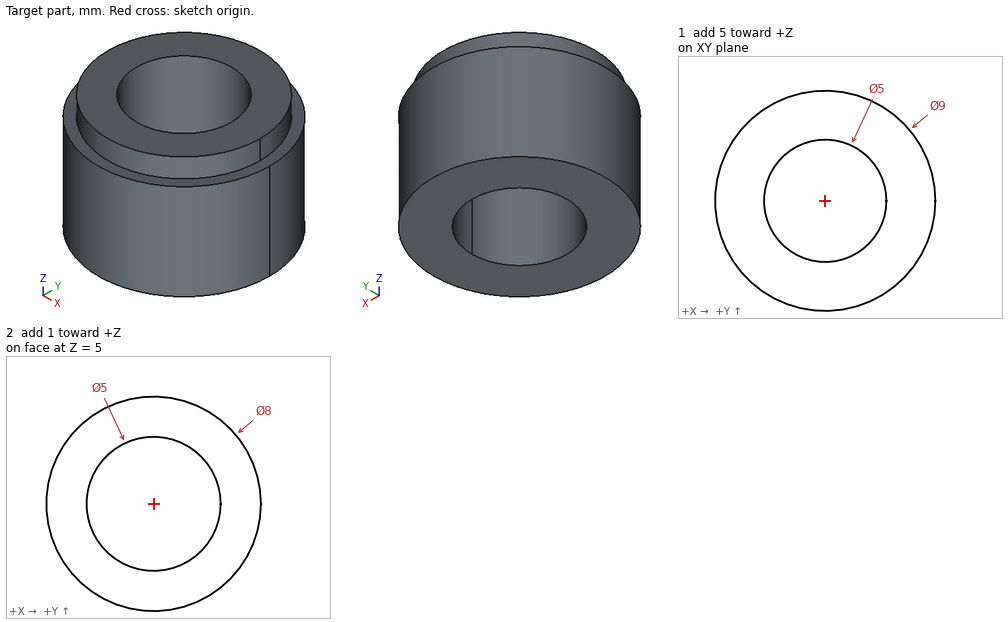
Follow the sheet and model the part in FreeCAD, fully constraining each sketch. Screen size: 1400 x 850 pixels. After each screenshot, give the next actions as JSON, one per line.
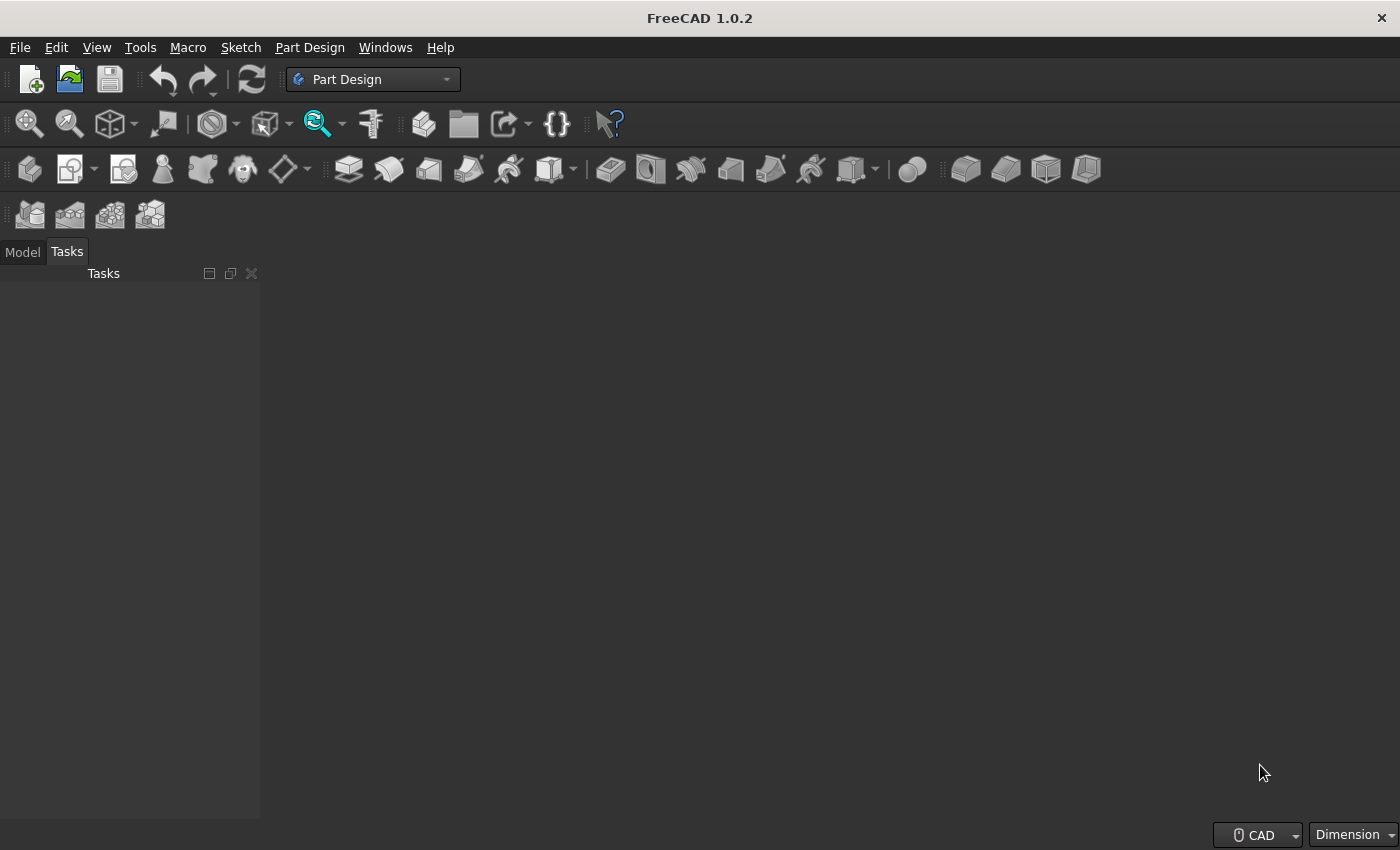
{"action": "left_click", "coordinate": [30, 80]}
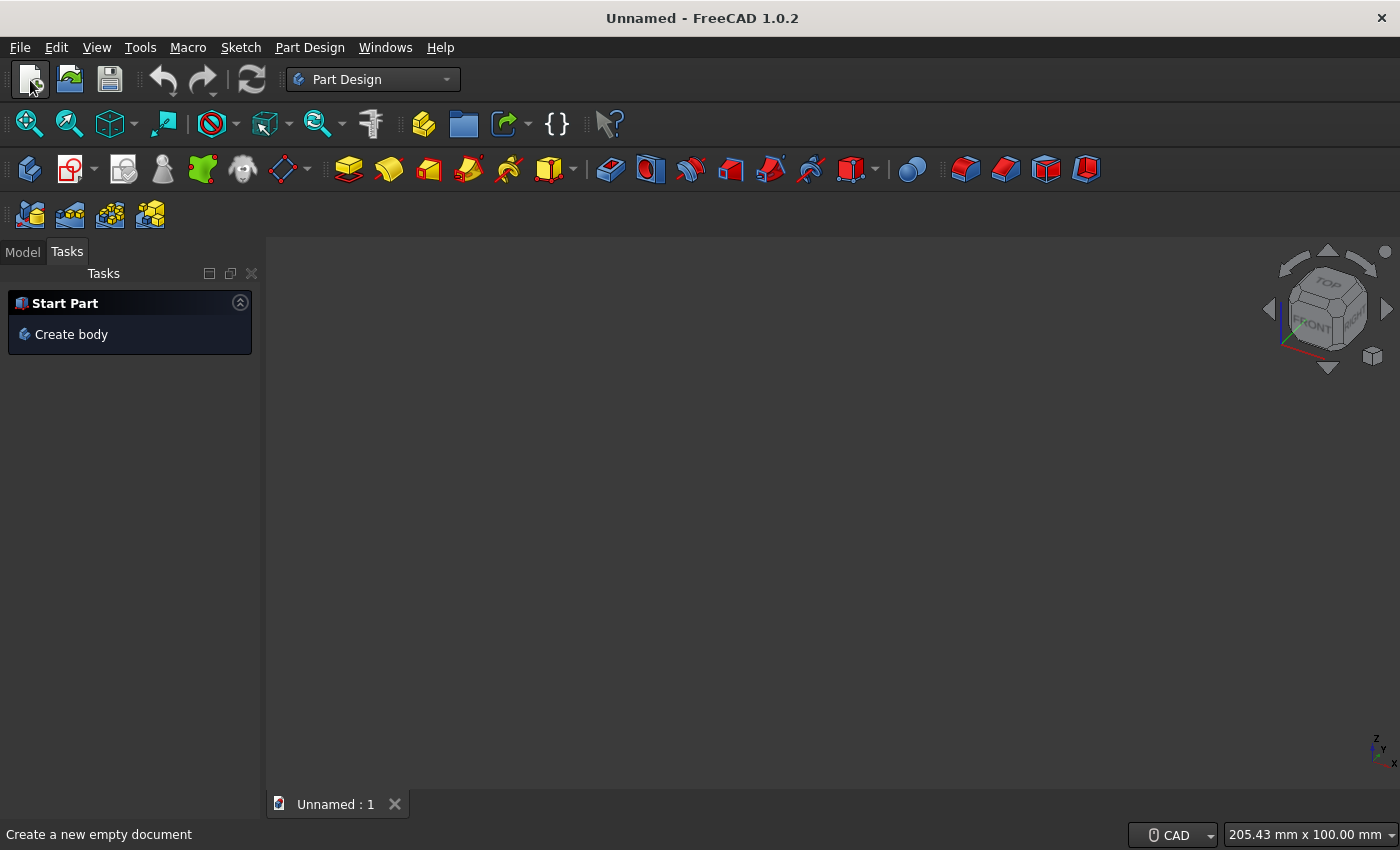
{"action": "left_click", "coordinate": [70, 170]}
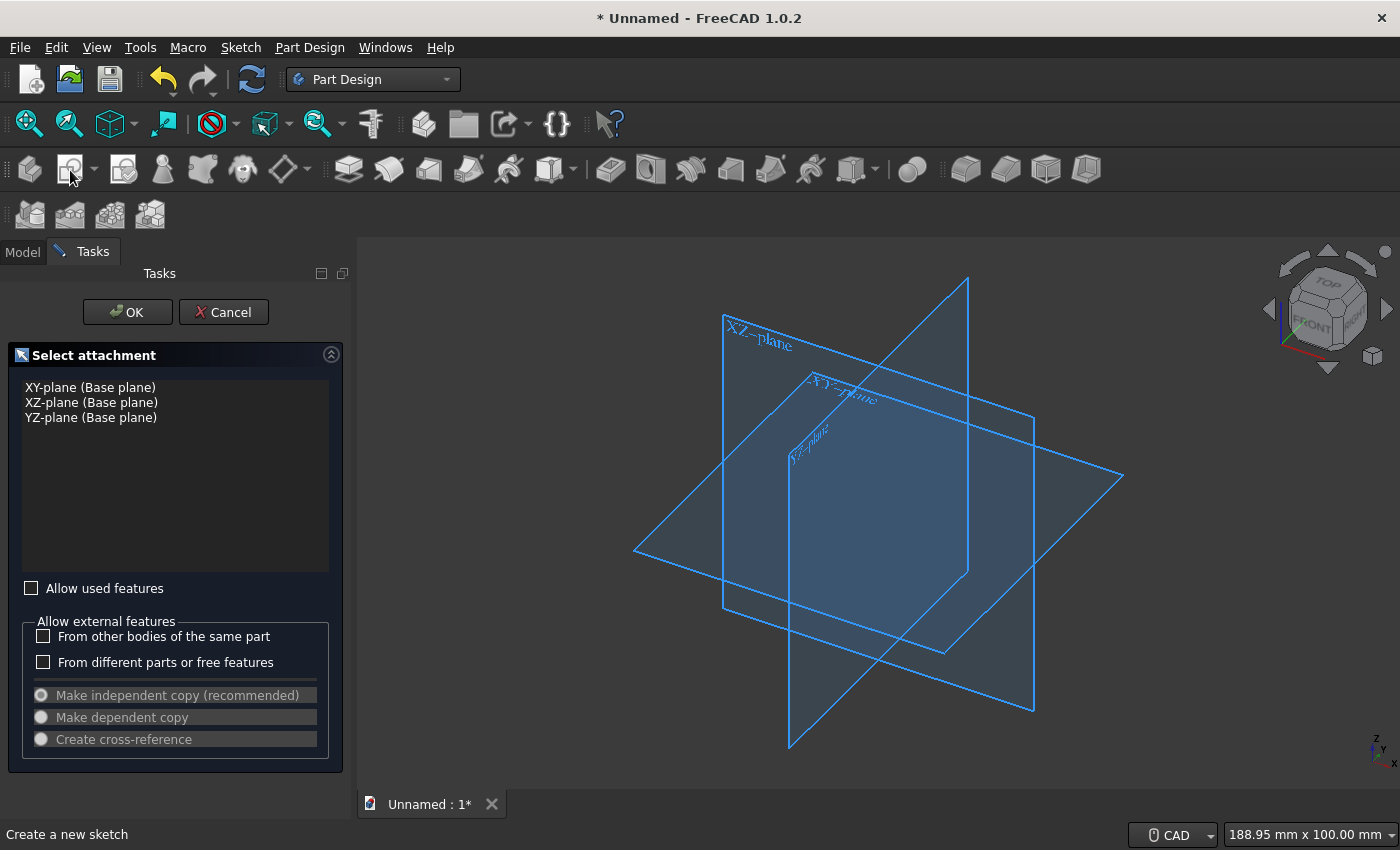
{"action": "left_click", "coordinate": [82, 388]}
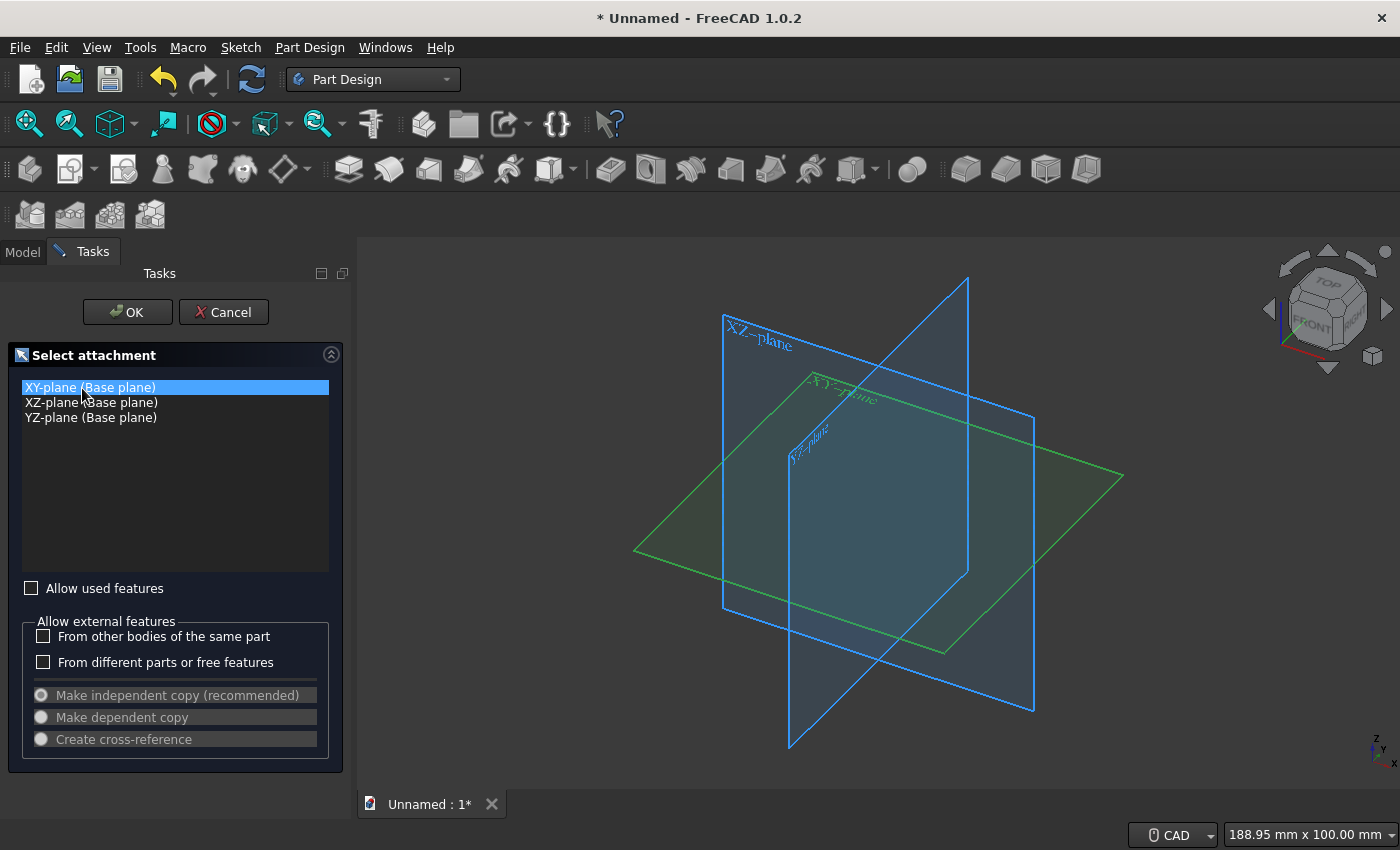
{"action": "left_click", "coordinate": [128, 312]}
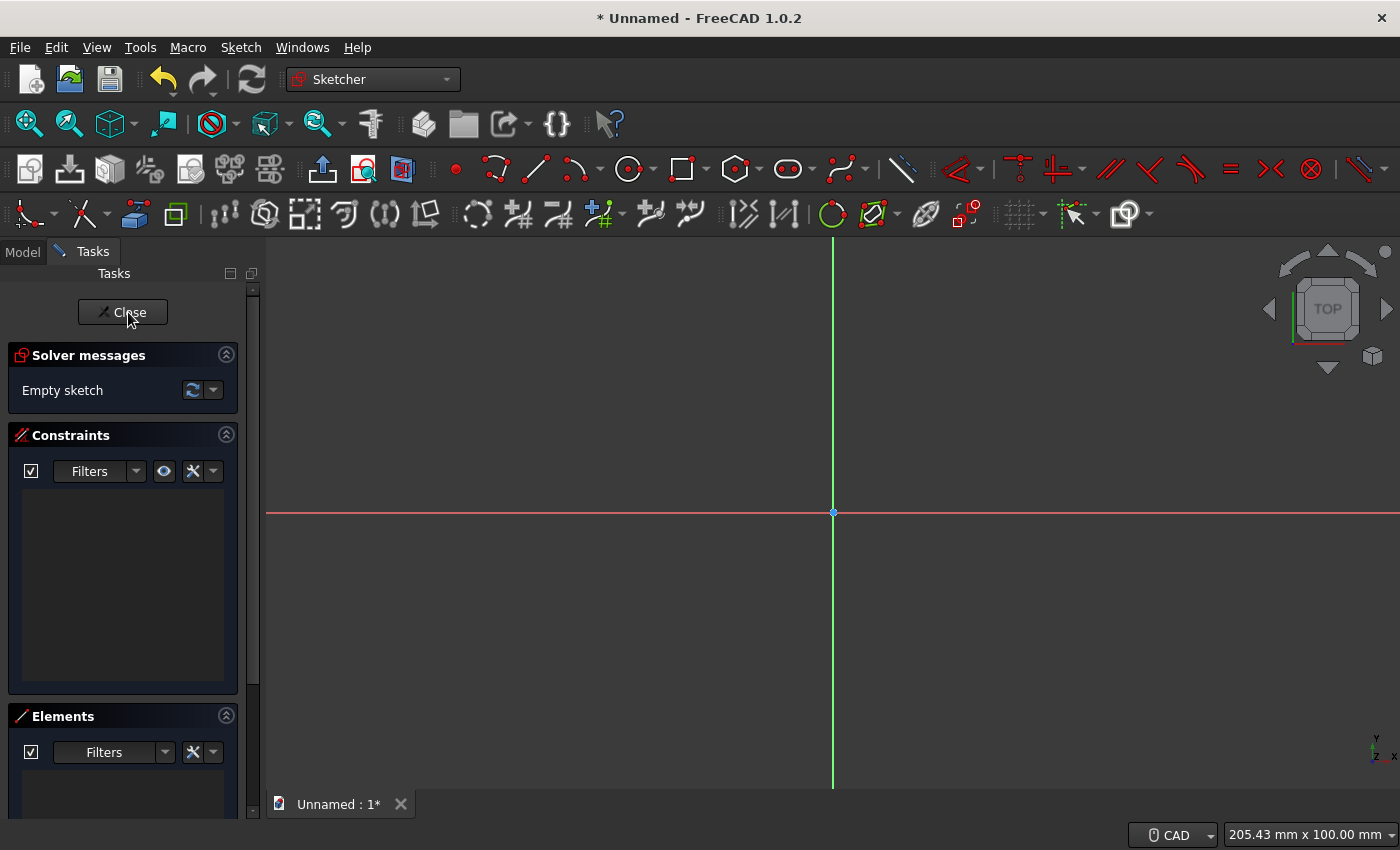
{"action": "scroll", "coordinate": [844, 513], "scroll_direction": "up", "scroll_amount": 10}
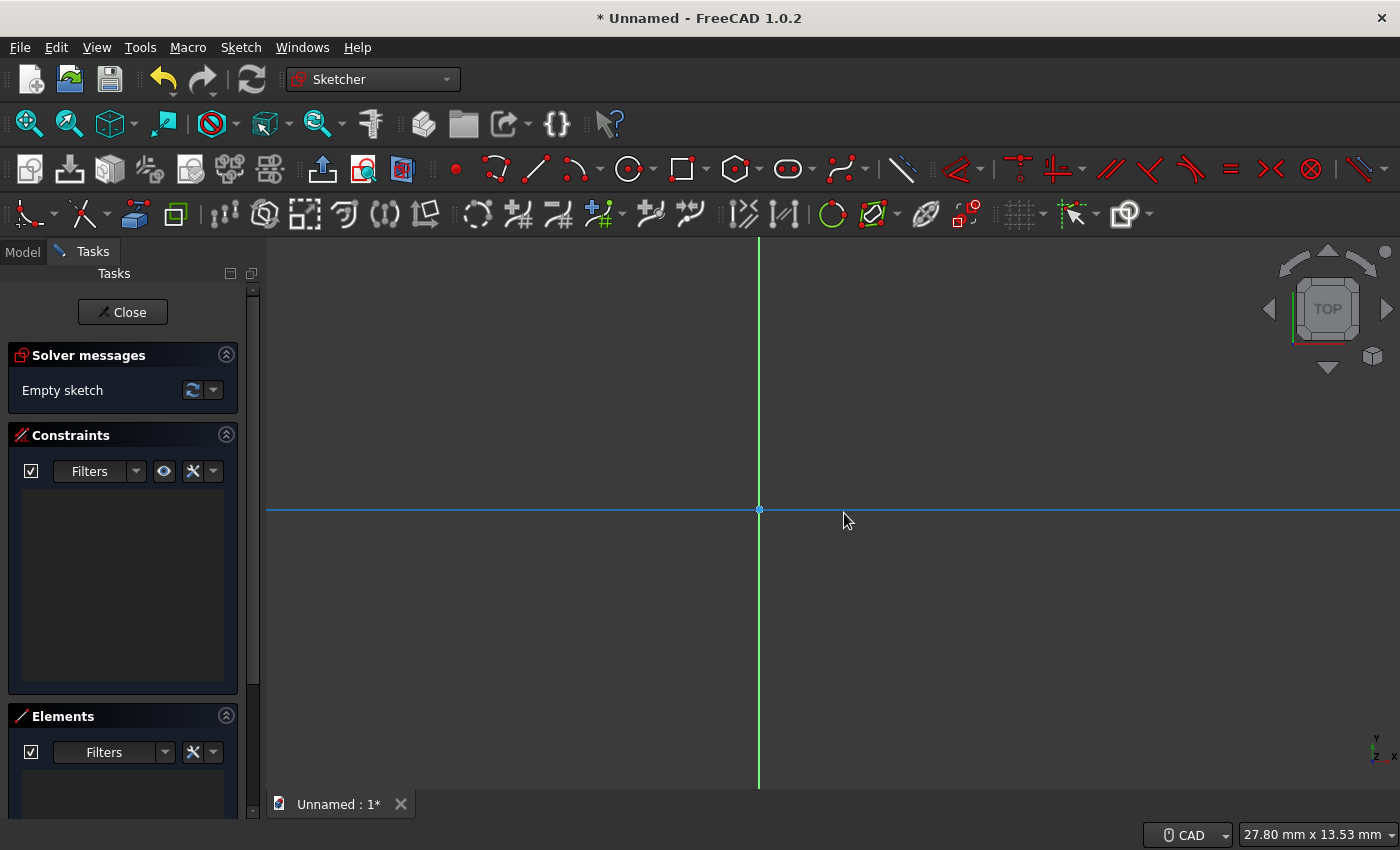
{"action": "left_click", "coordinate": [630, 170]}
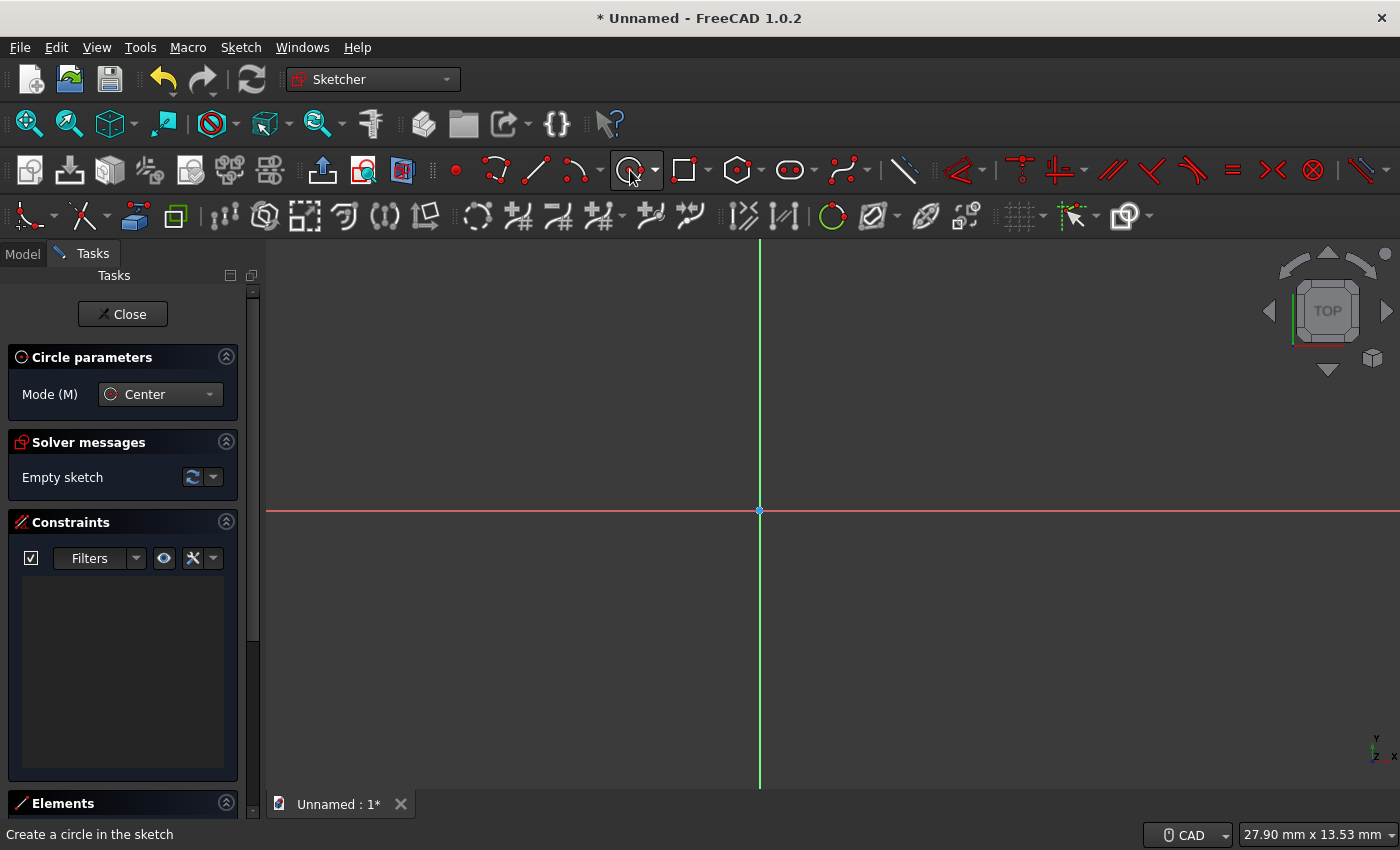
{"action": "left_click", "coordinate": [760, 511]}
{"action": "left_click", "coordinate": [889, 381]}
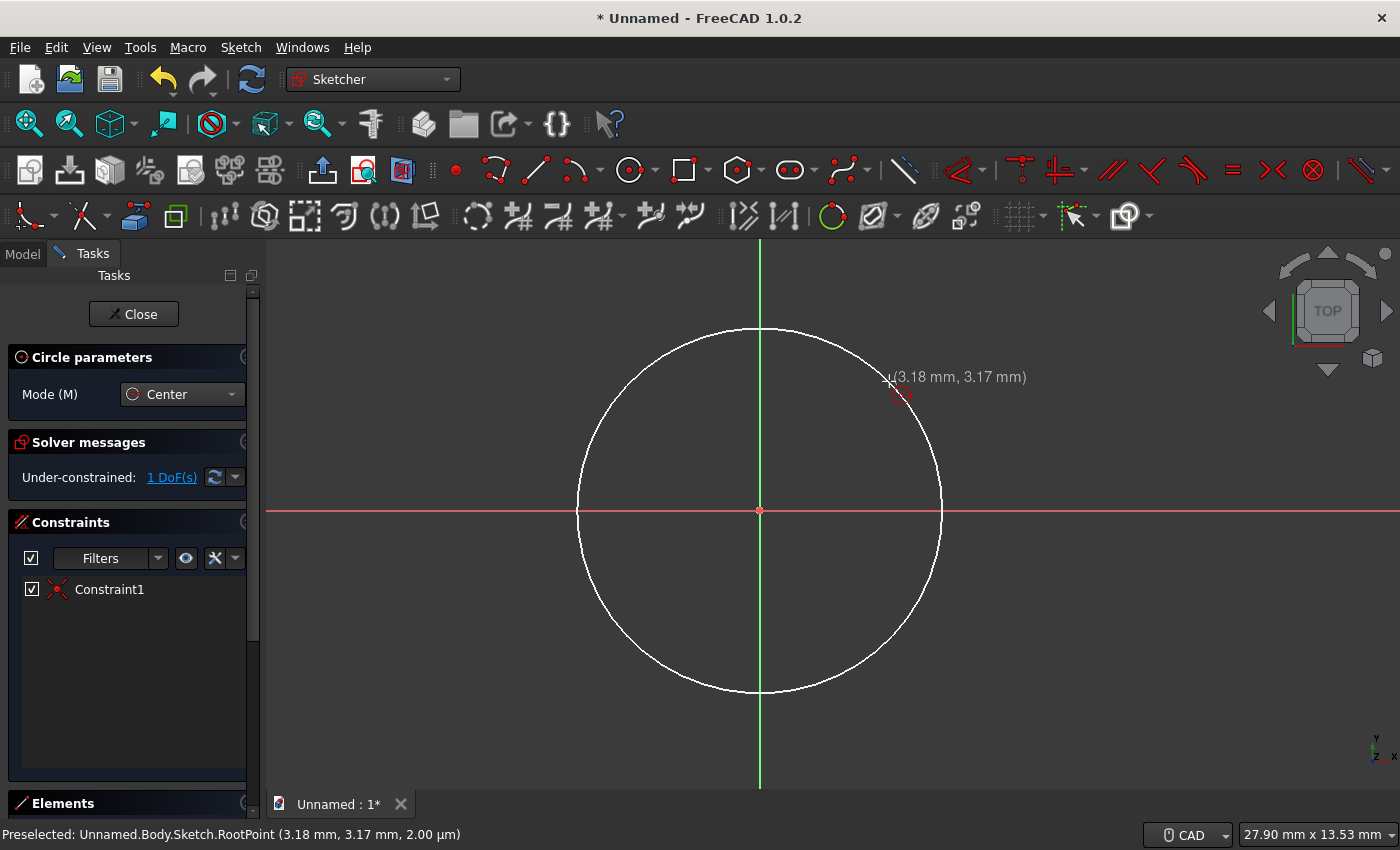
{"action": "left_click", "coordinate": [760, 511]}
{"action": "left_click", "coordinate": [832, 439]}
{"action": "key", "text": "Escape"}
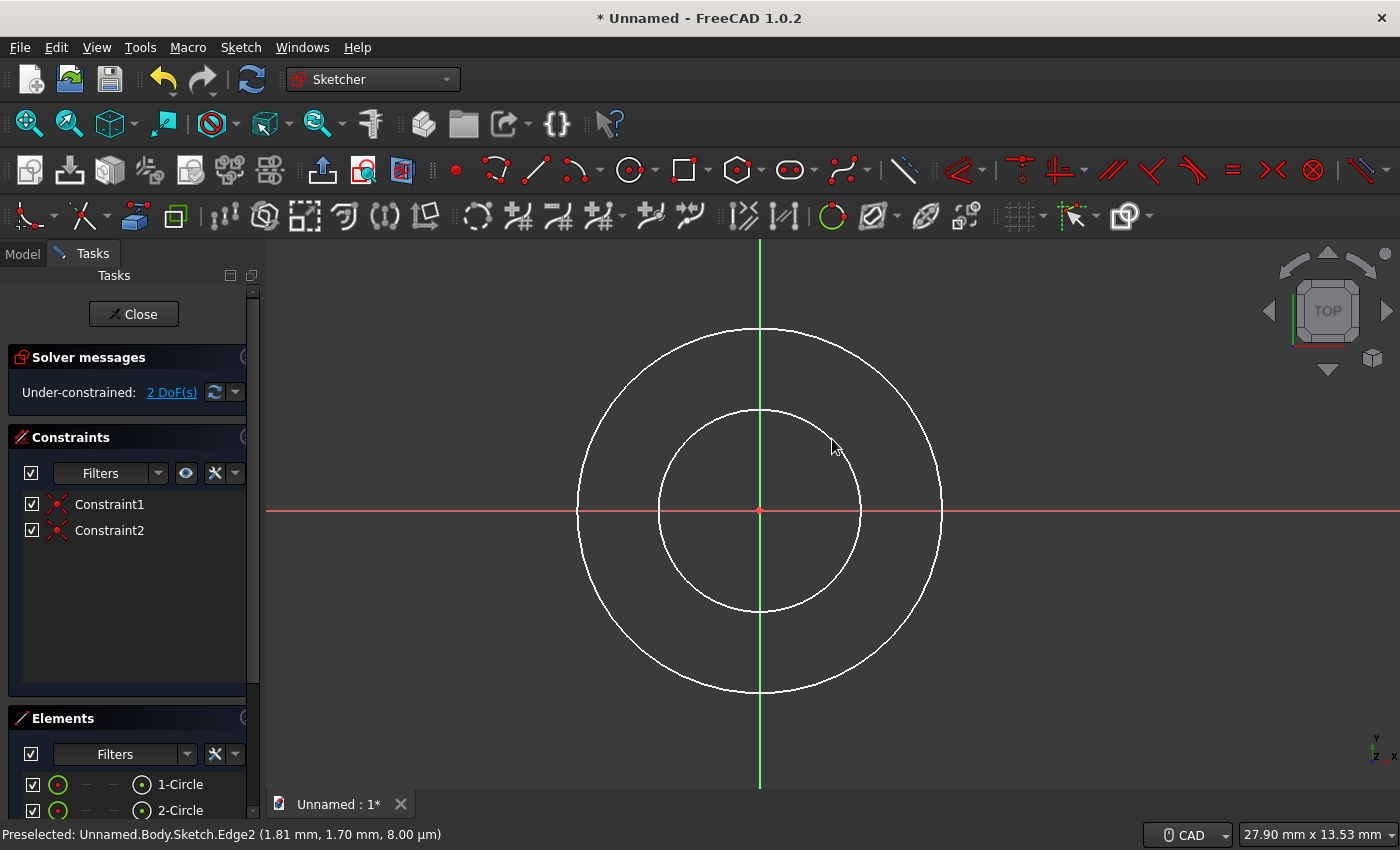
{"action": "left_click", "coordinate": [958, 170]}